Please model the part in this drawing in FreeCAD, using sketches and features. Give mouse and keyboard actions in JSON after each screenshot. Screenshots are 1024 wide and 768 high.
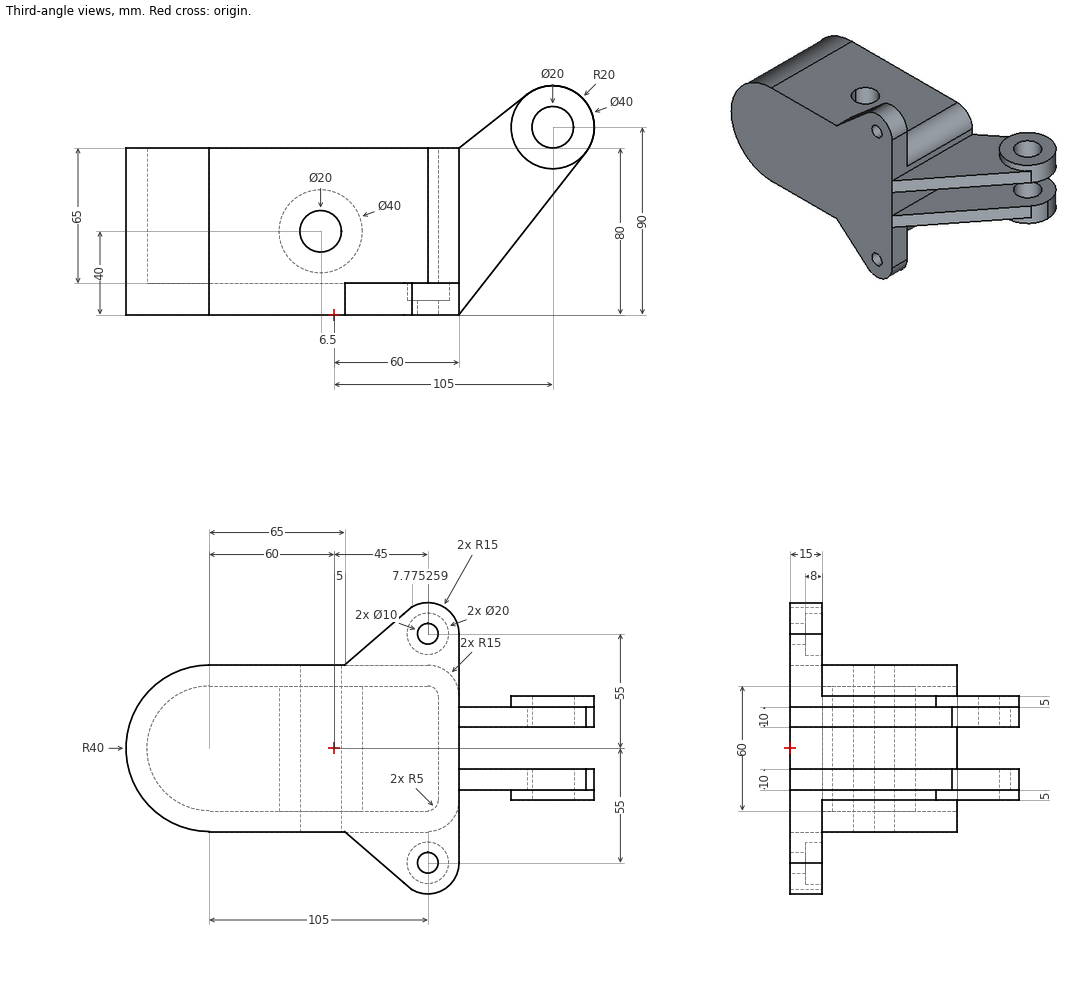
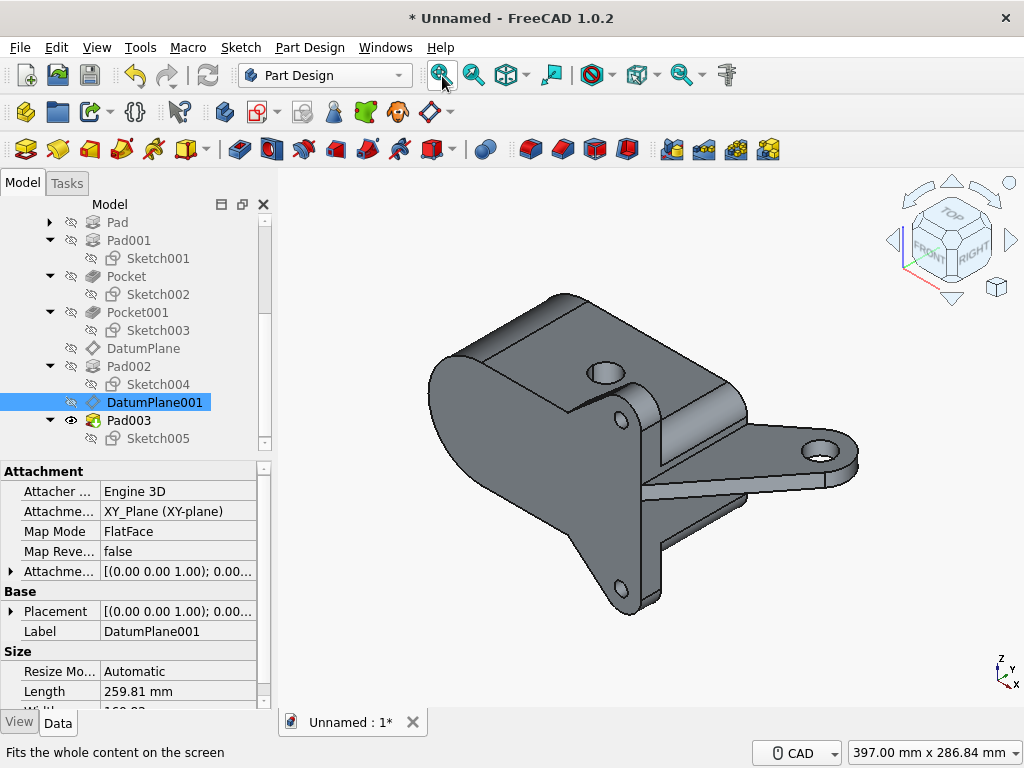
{"action": "left_click", "coordinate": [766, 448]}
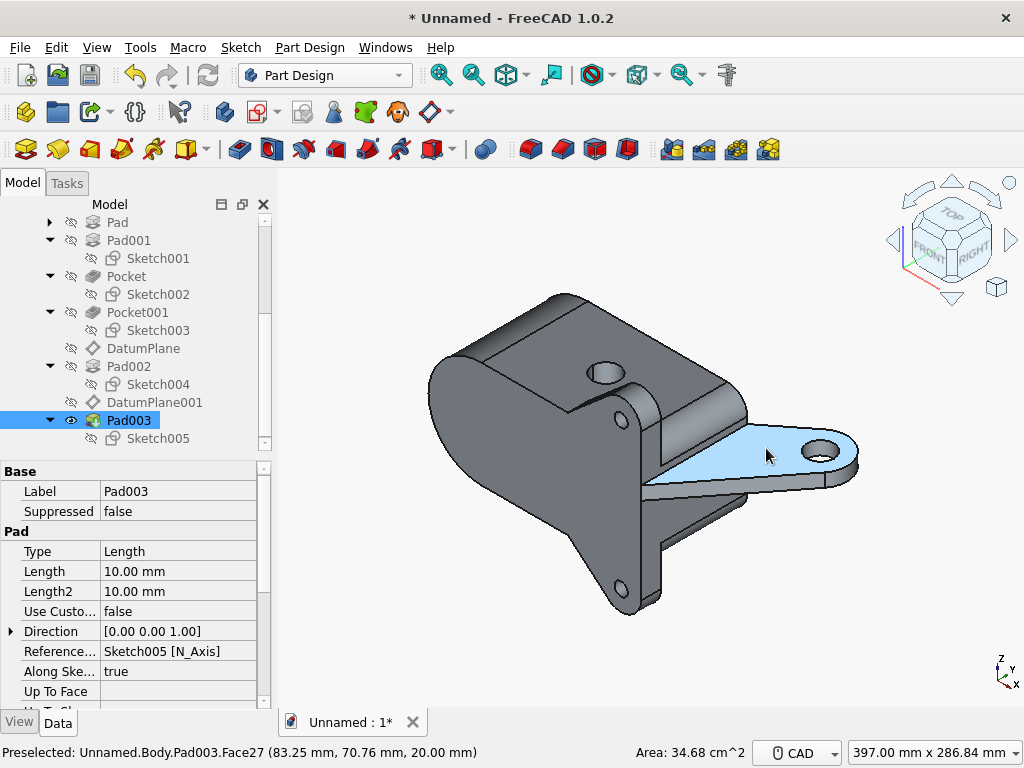
{"action": "left_click", "coordinate": [258, 112]}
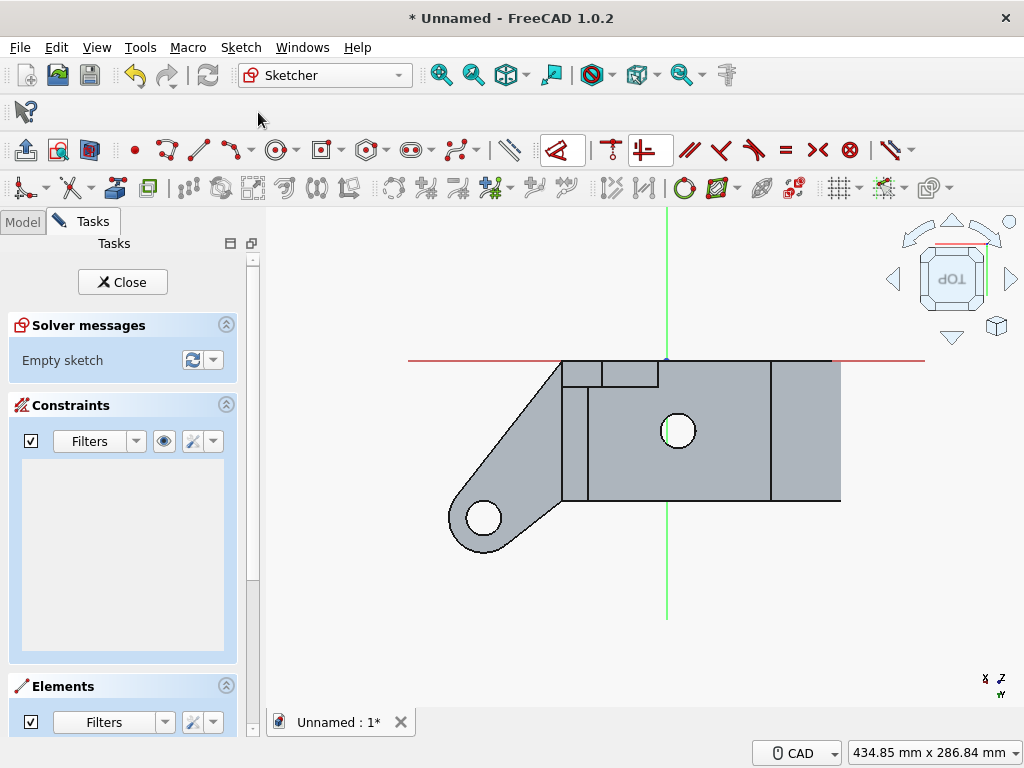
{"action": "scroll", "coordinate": [460, 533], "scroll_direction": "up", "scroll_amount": 8}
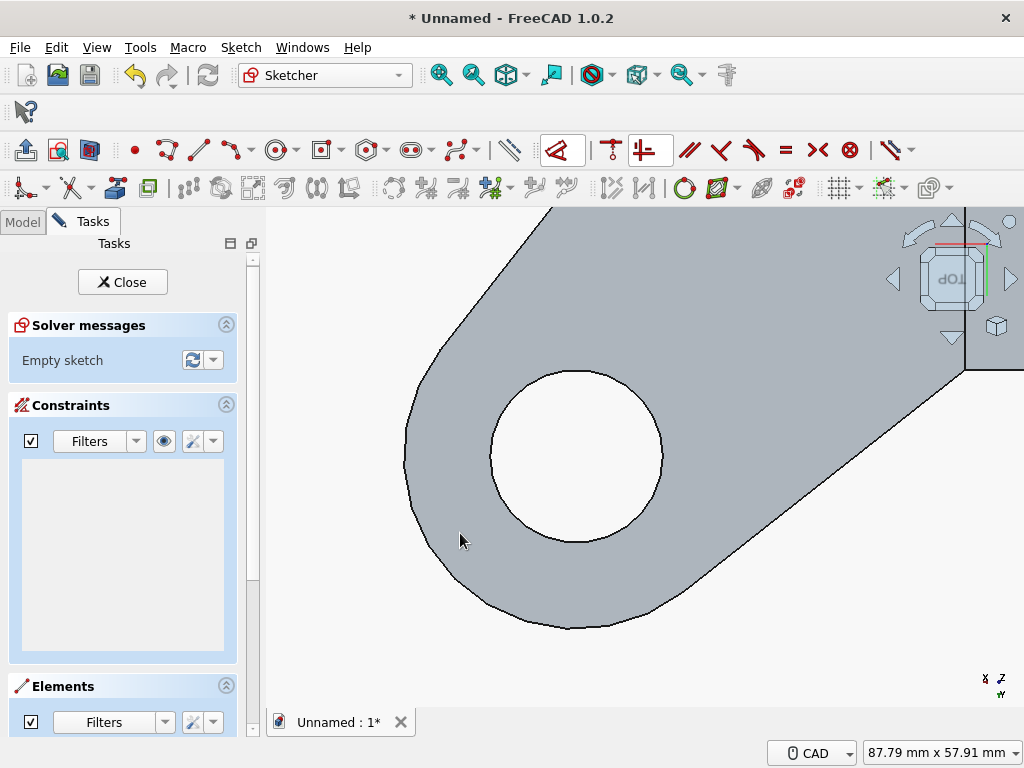
{"action": "left_click", "coordinate": [276, 150]}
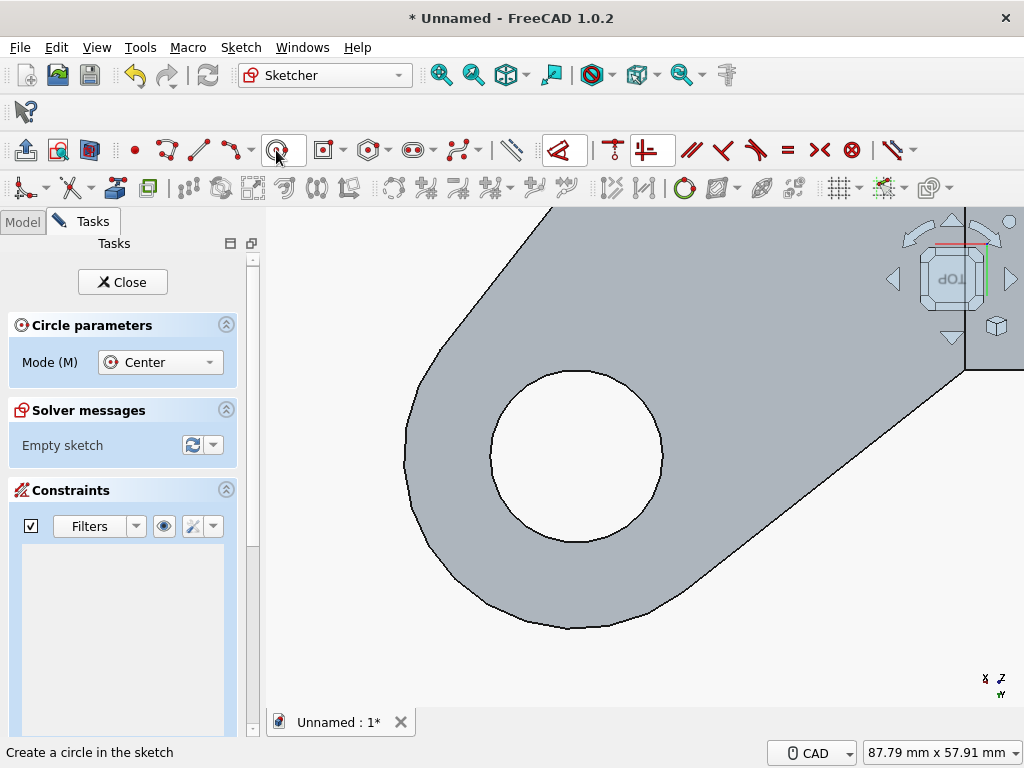
{"action": "left_click", "coordinate": [577, 456]}
{"action": "left_click", "coordinate": [699, 334]}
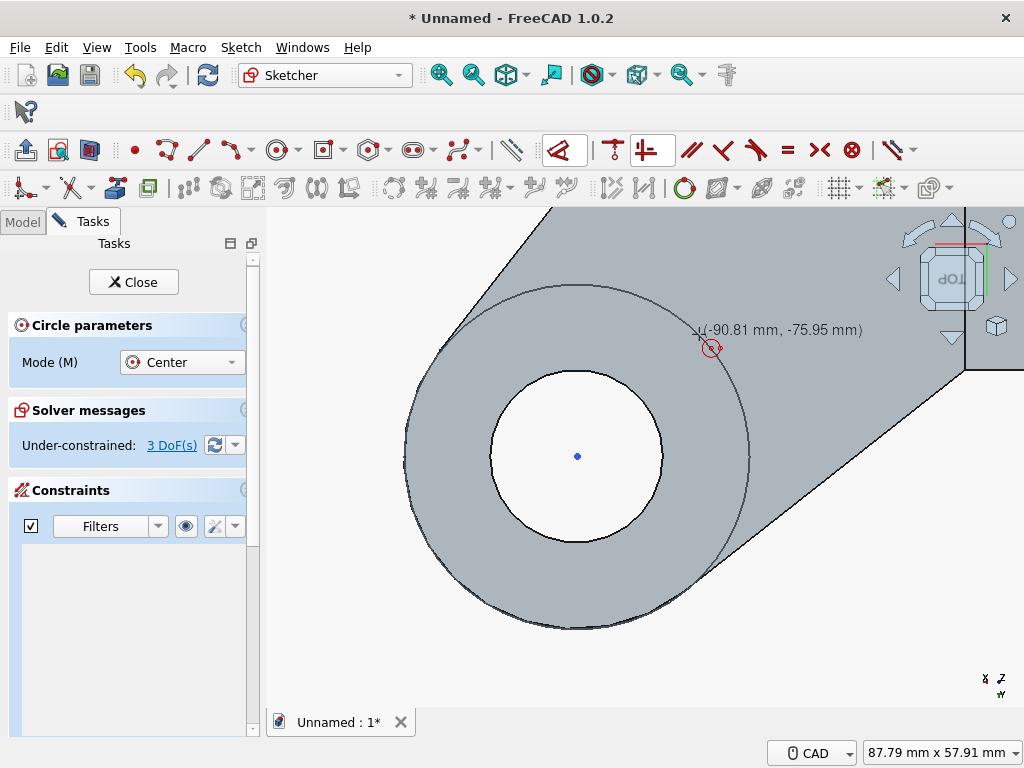
{"action": "left_click", "coordinate": [577, 457]}
{"action": "left_click", "coordinate": [638, 395]}
{"action": "key", "text": "Escape"}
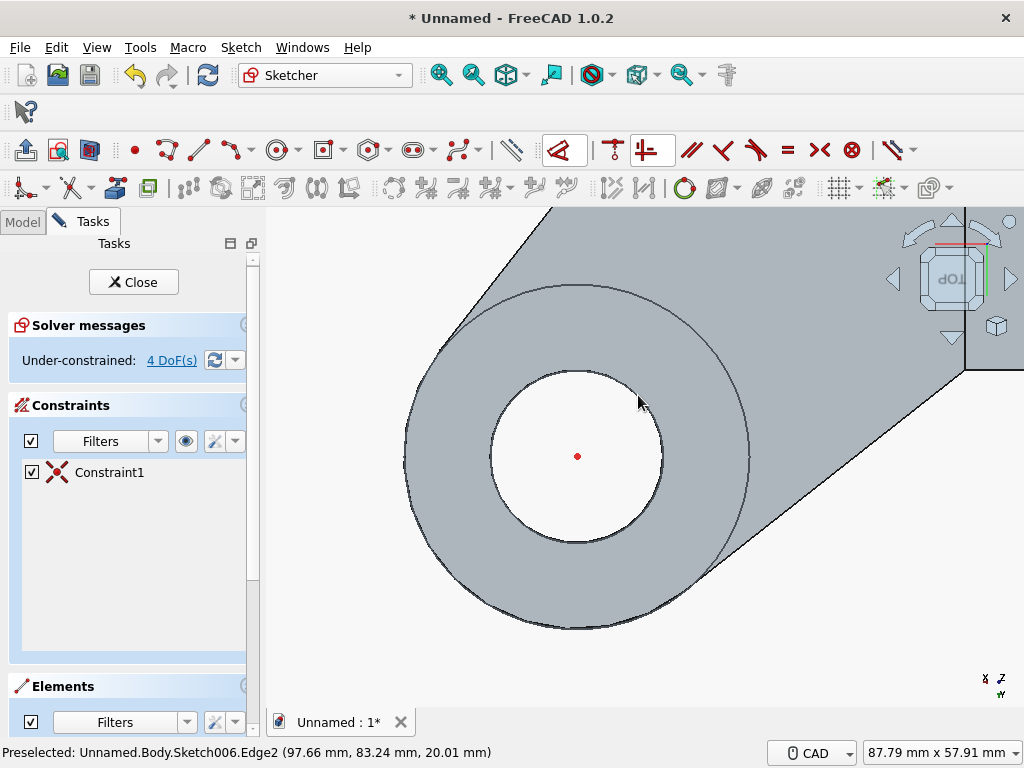
{"action": "left_click", "coordinate": [699, 335]}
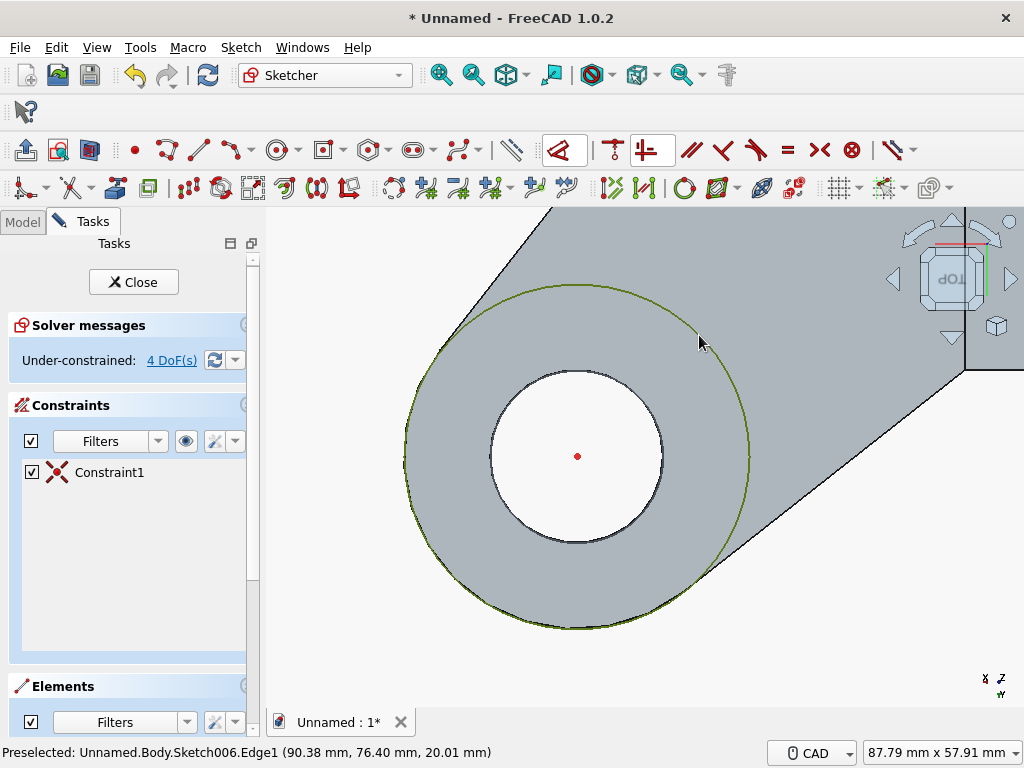
{"action": "key", "text": "k o"}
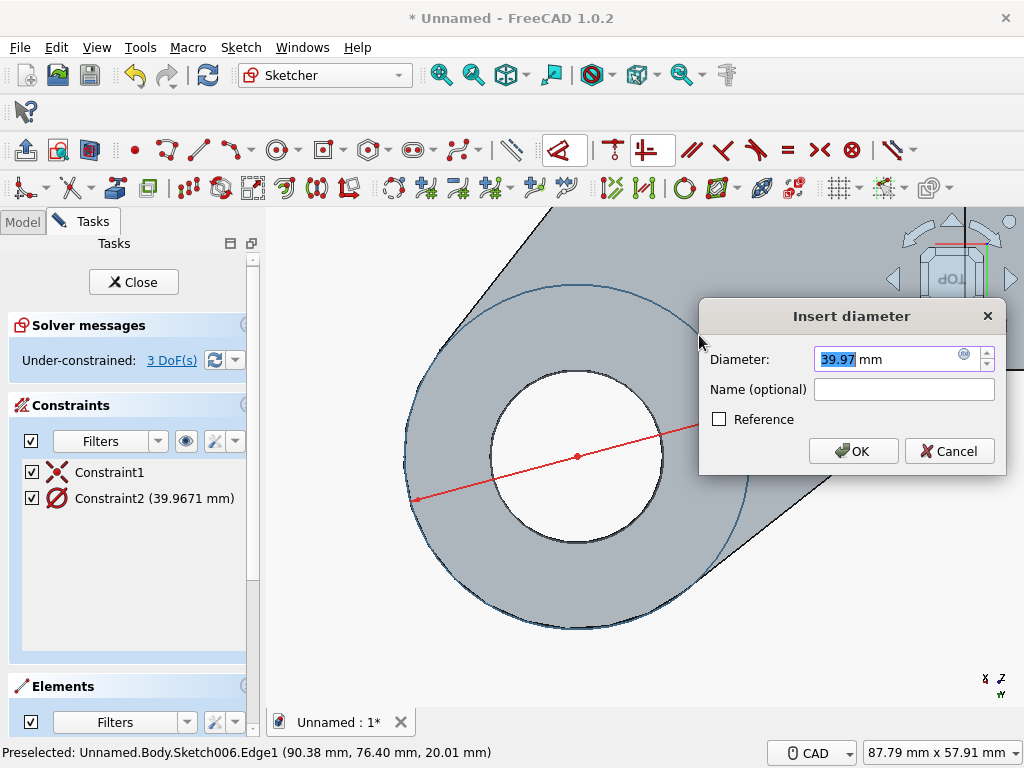
{"action": "type", "text": "40"}
{"action": "key", "text": "Return"}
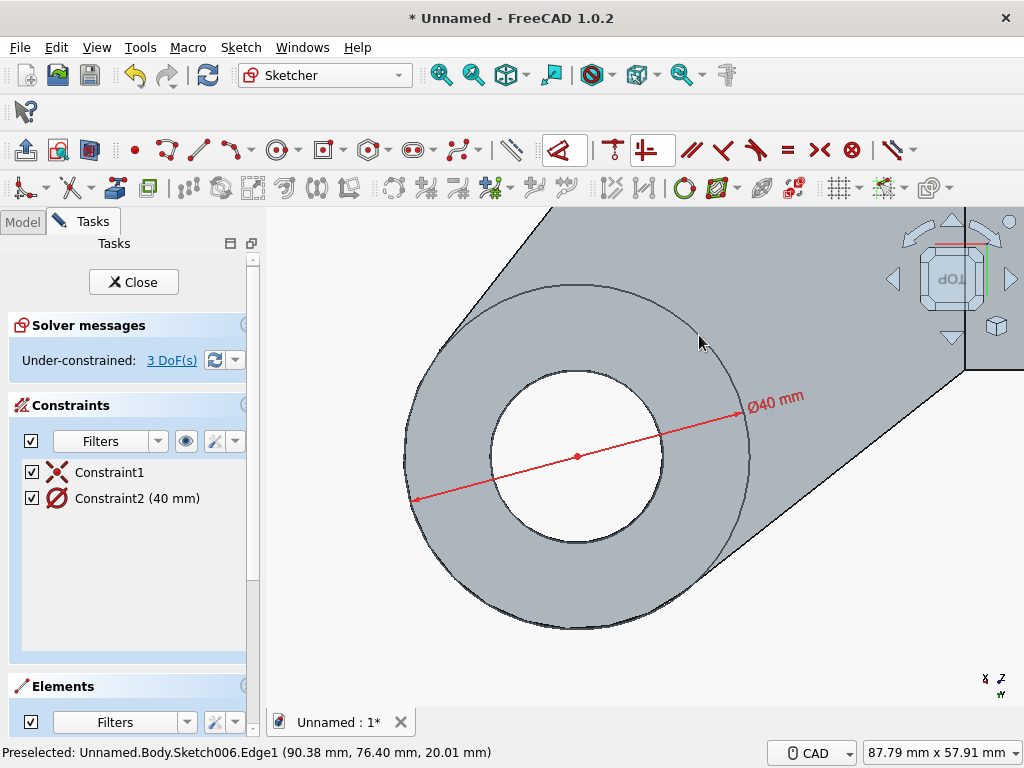
{"action": "left_click", "coordinate": [638, 396]}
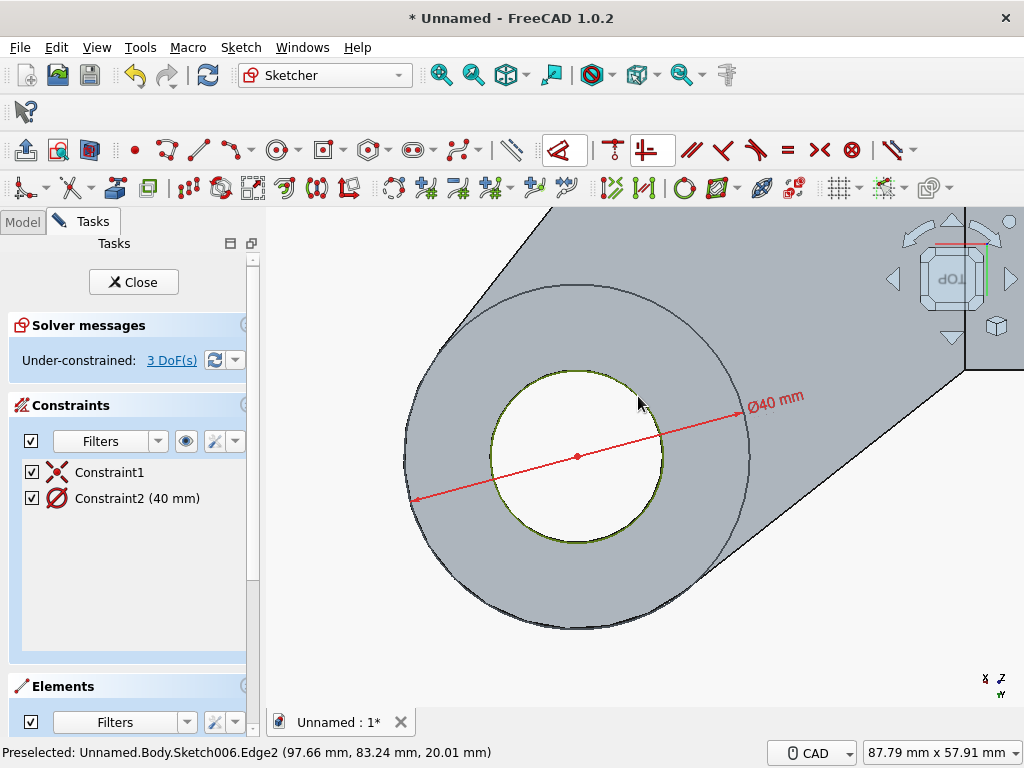
{"action": "left_click", "coordinate": [582, 150]}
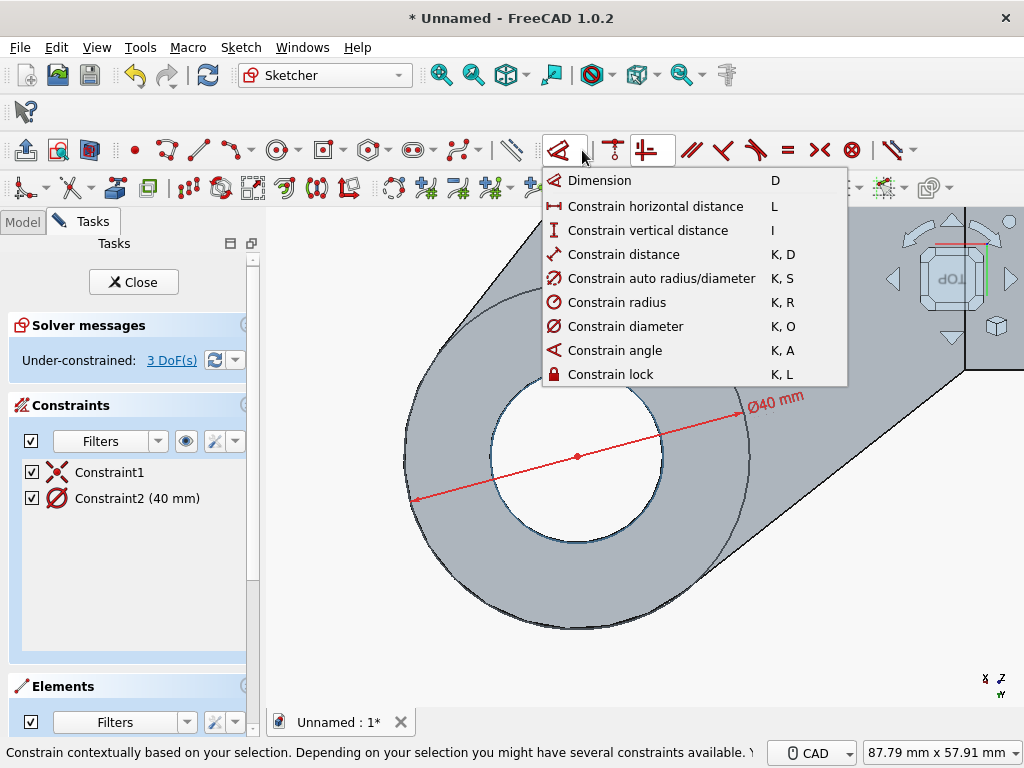
{"action": "left_click", "coordinate": [695, 326]}